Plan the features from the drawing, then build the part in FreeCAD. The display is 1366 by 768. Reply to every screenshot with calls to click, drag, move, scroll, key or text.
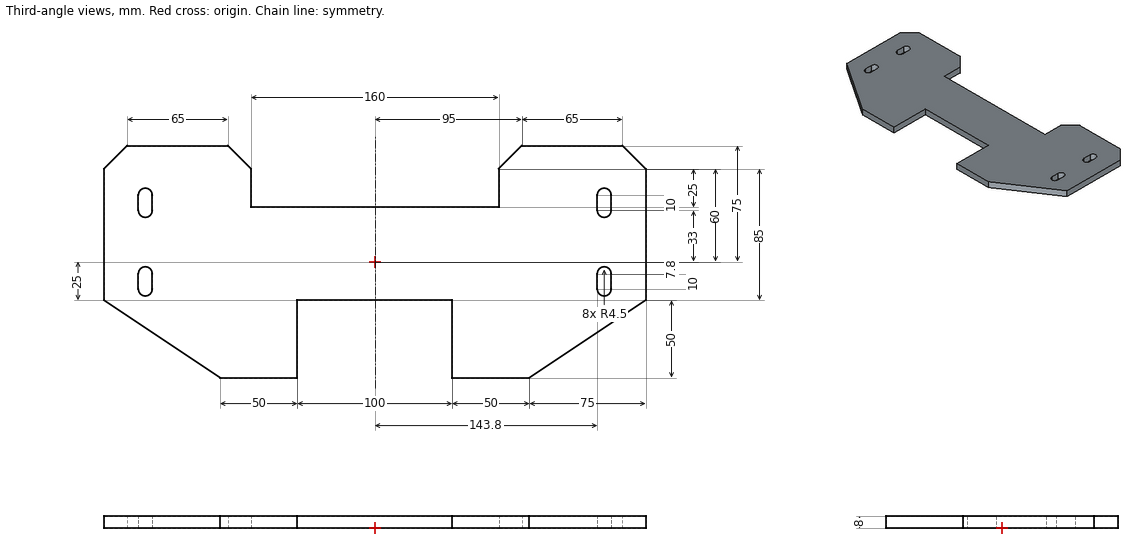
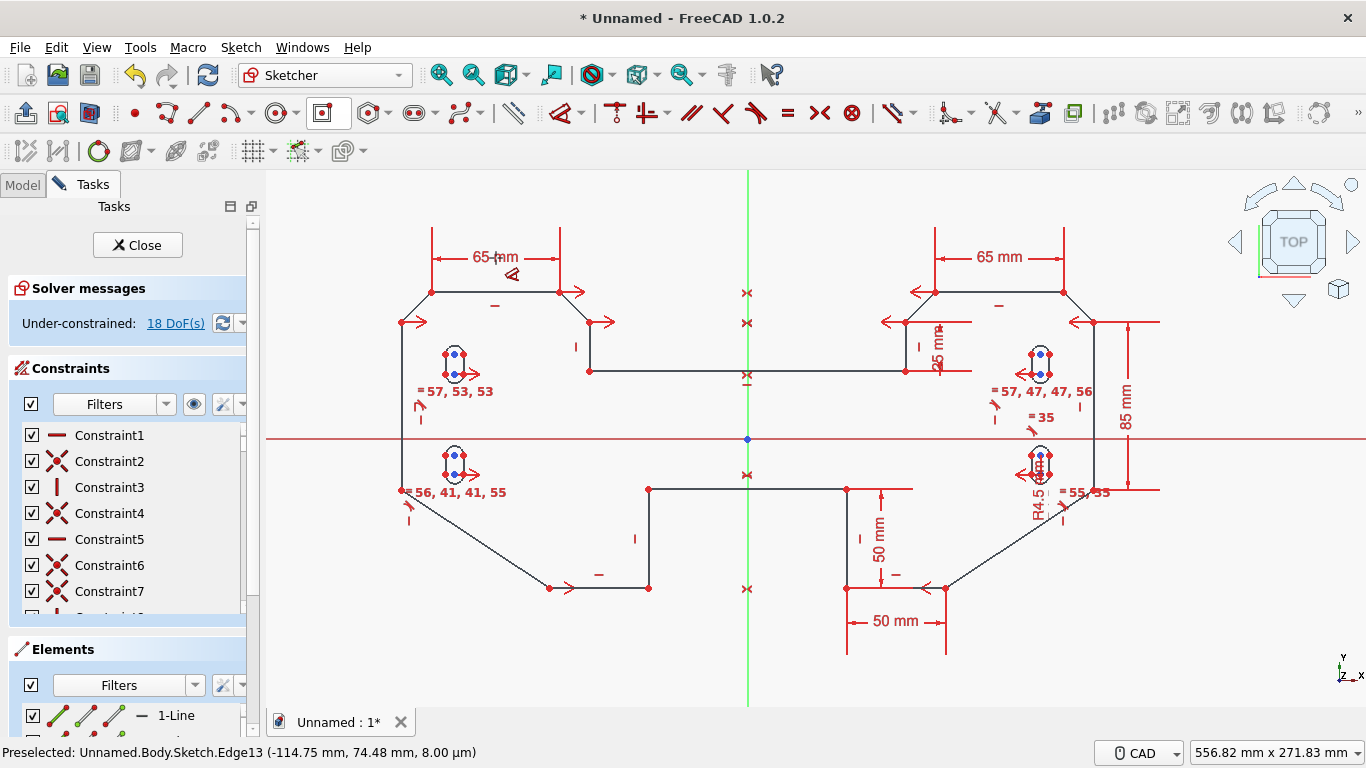
click(402, 373)
click(368, 406)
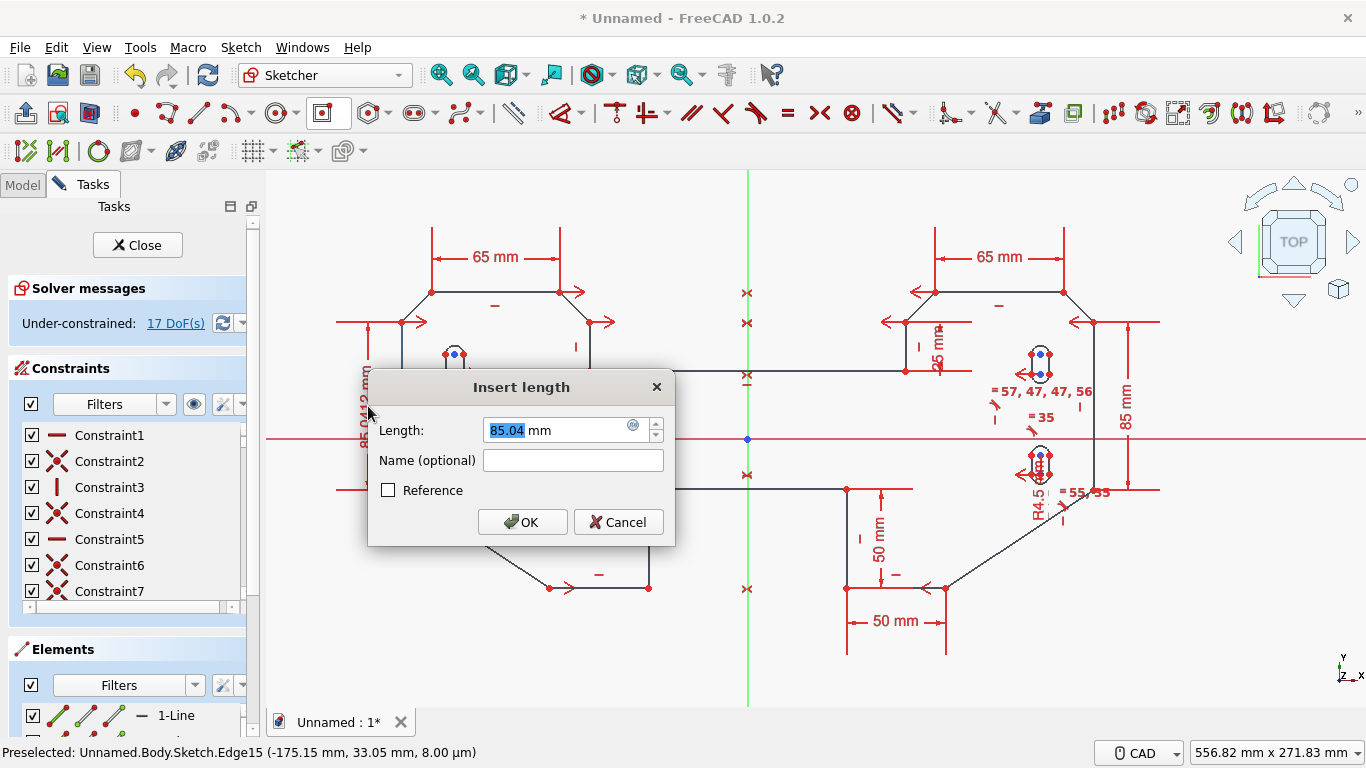
text(85)
key(Return)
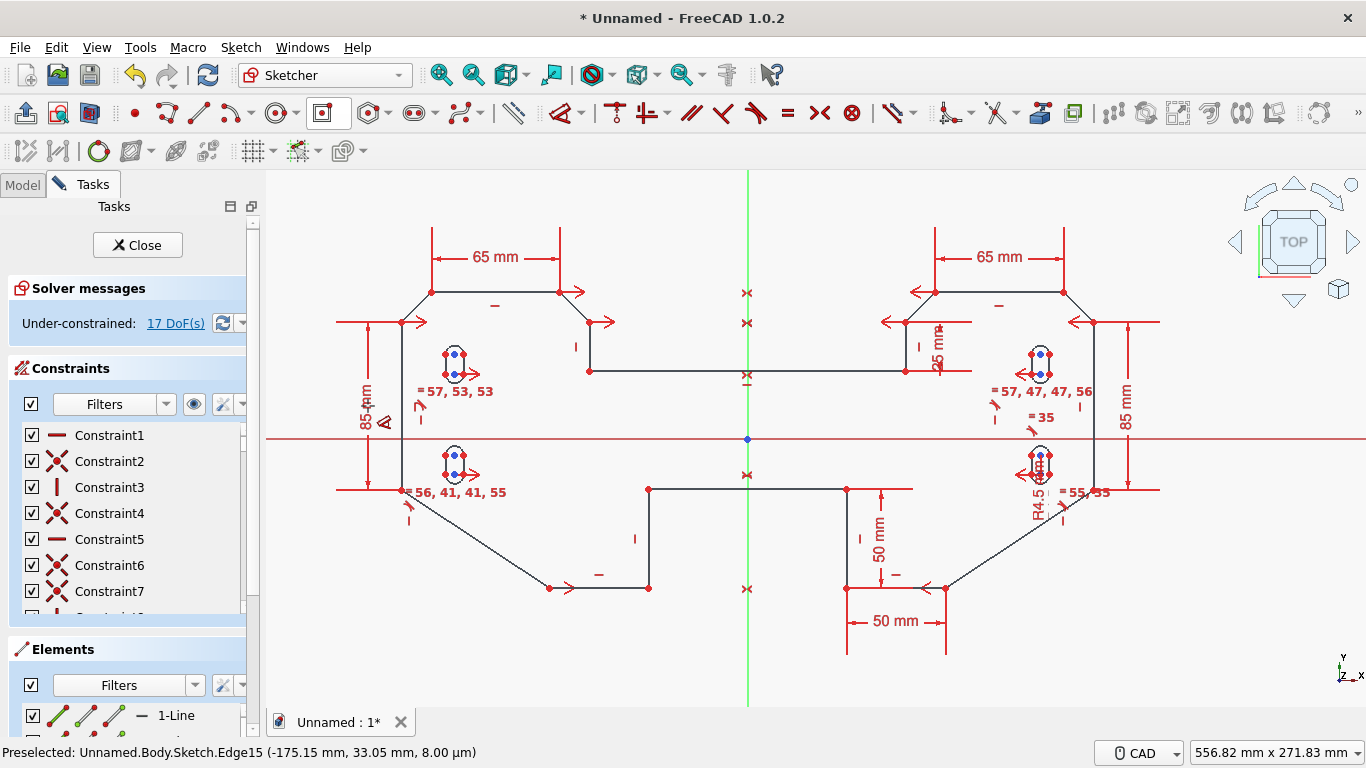
click(579, 588)
click(599, 622)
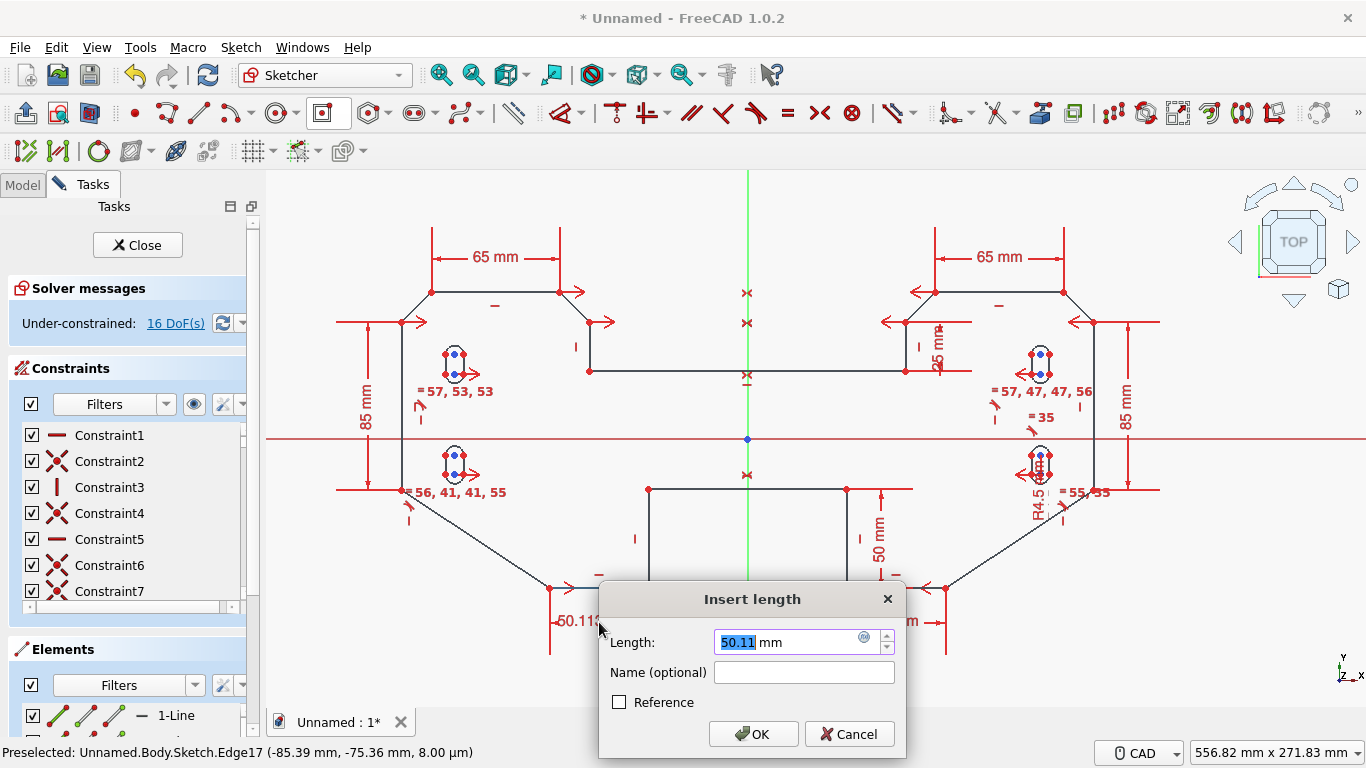
text(50)
key(Return)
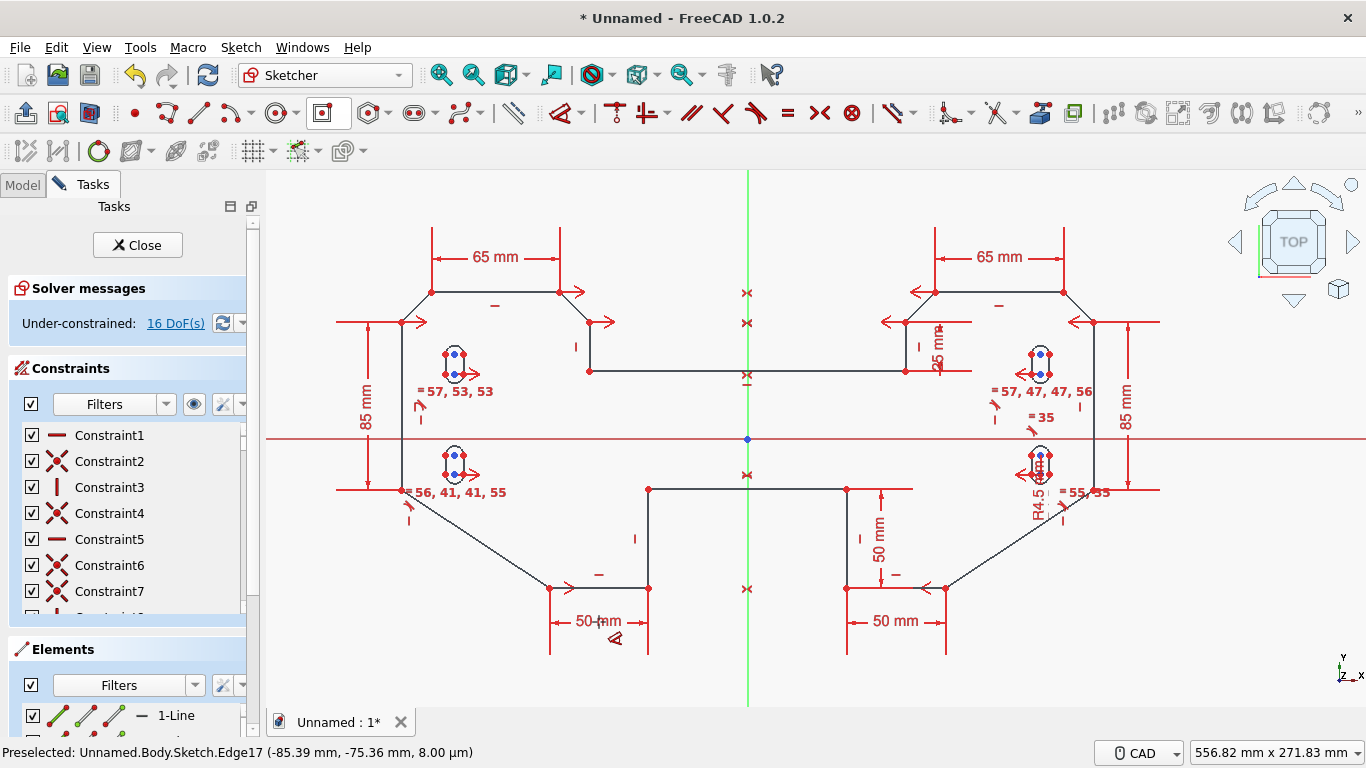
scroll(1032, 465, up, 4)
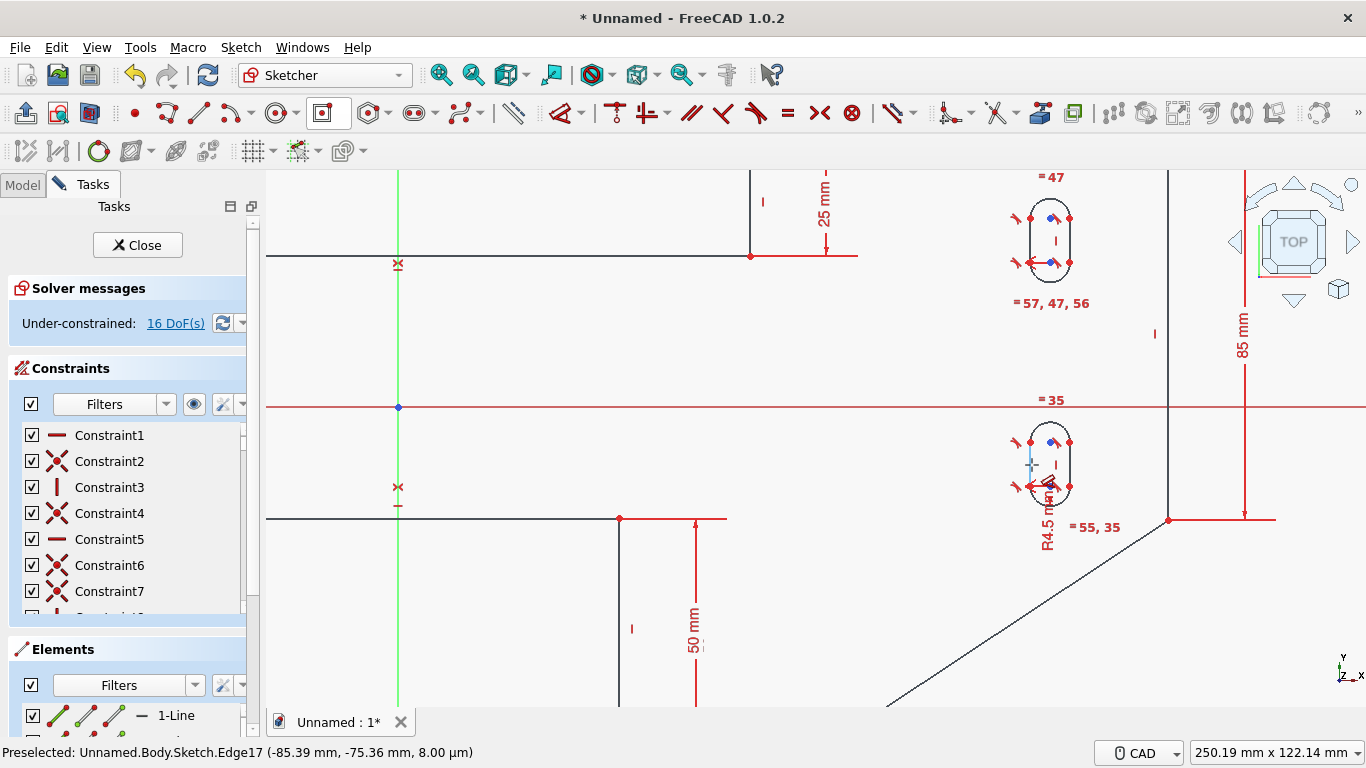
click(1030, 464)
click(996, 464)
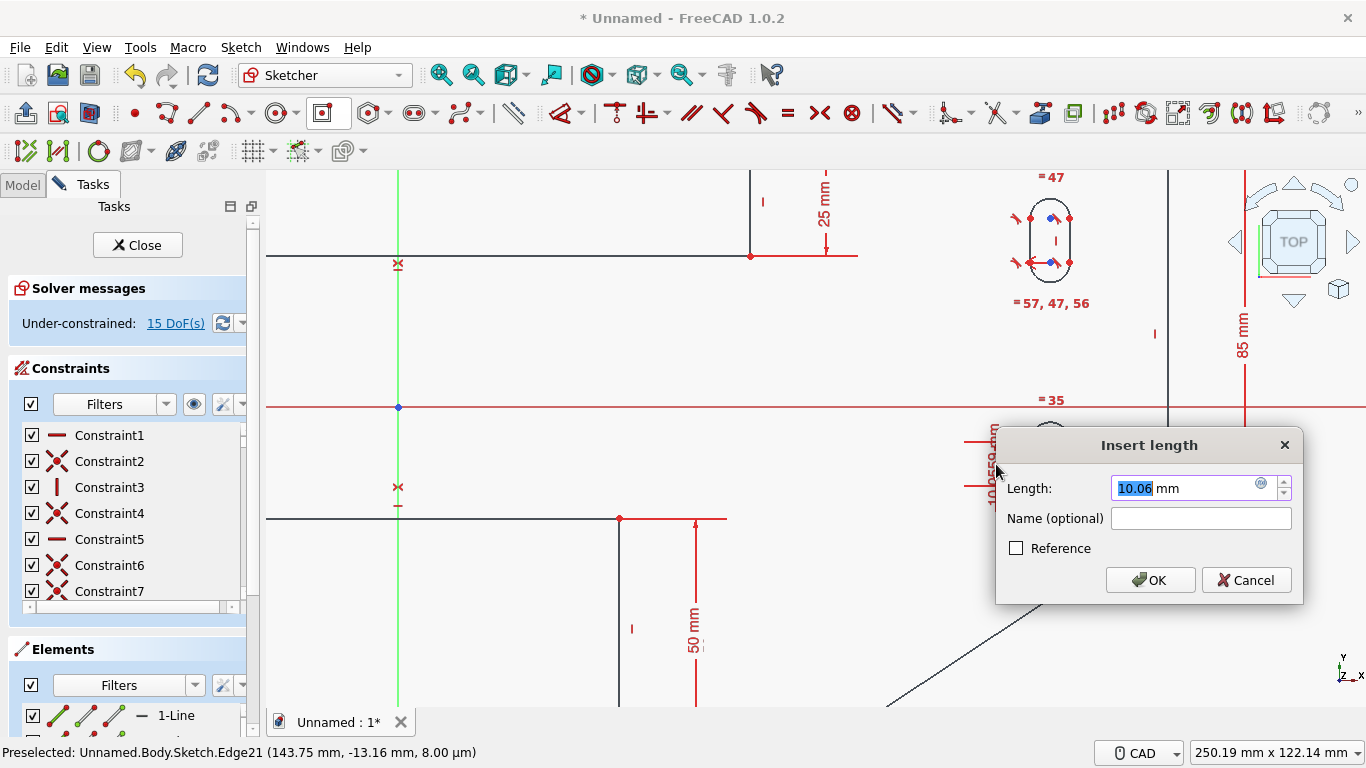
text(10)
key(Return)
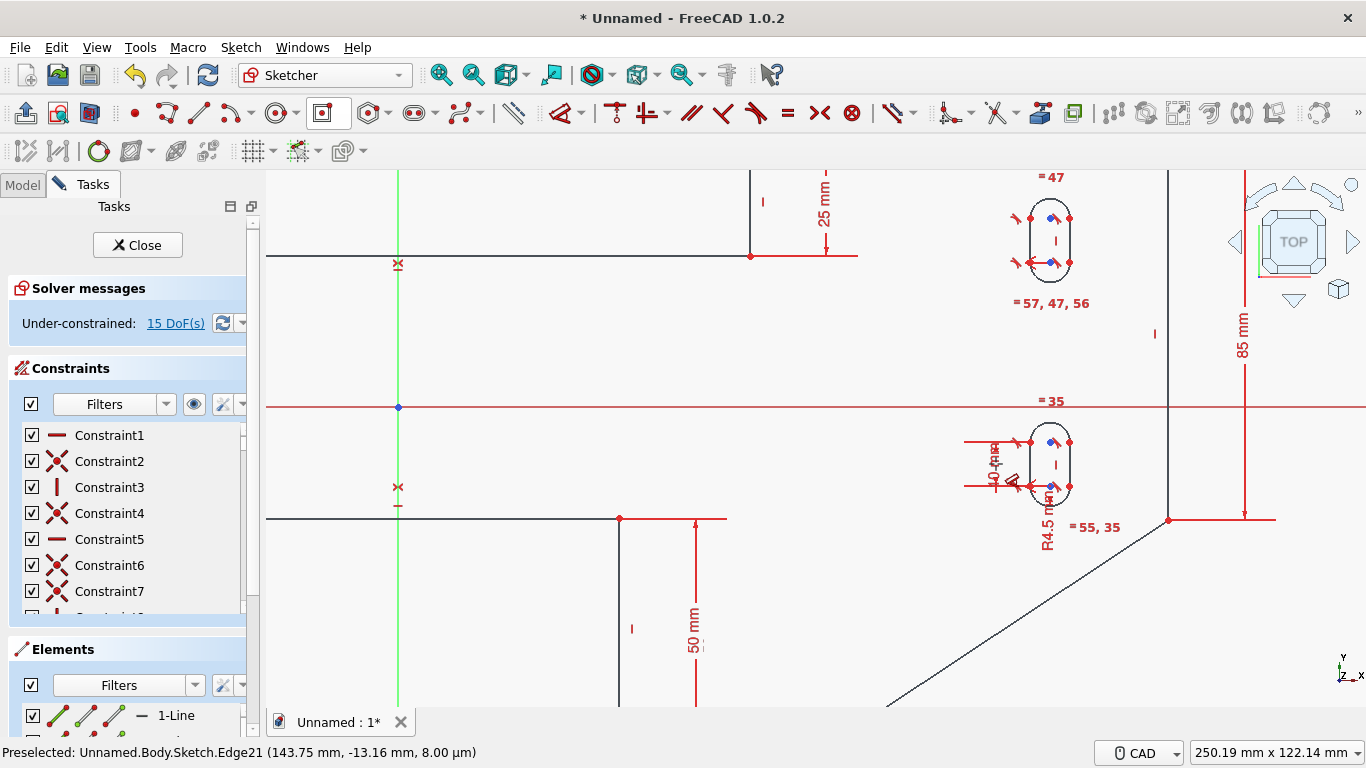
scroll(1032, 464, down, 4)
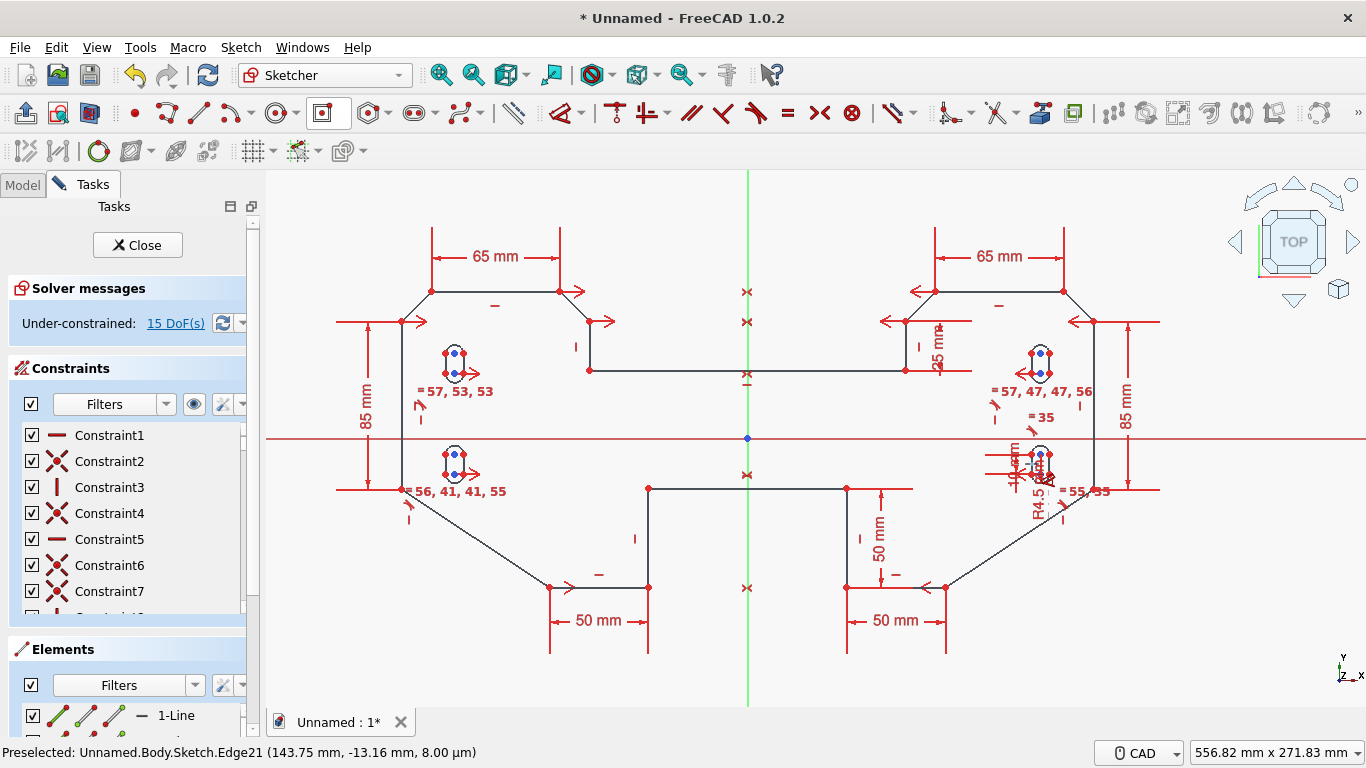
scroll(446, 468, up, 5)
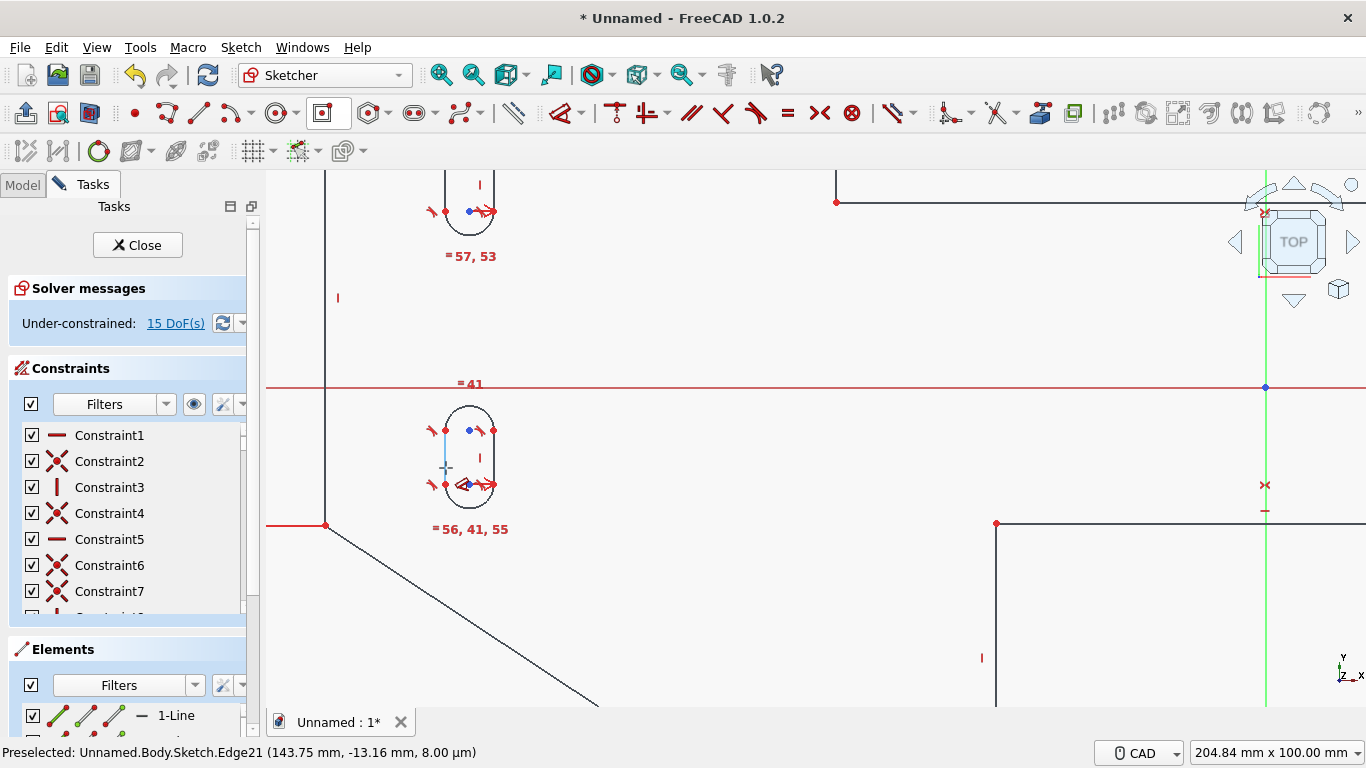
click(445, 468)
click(411, 457)